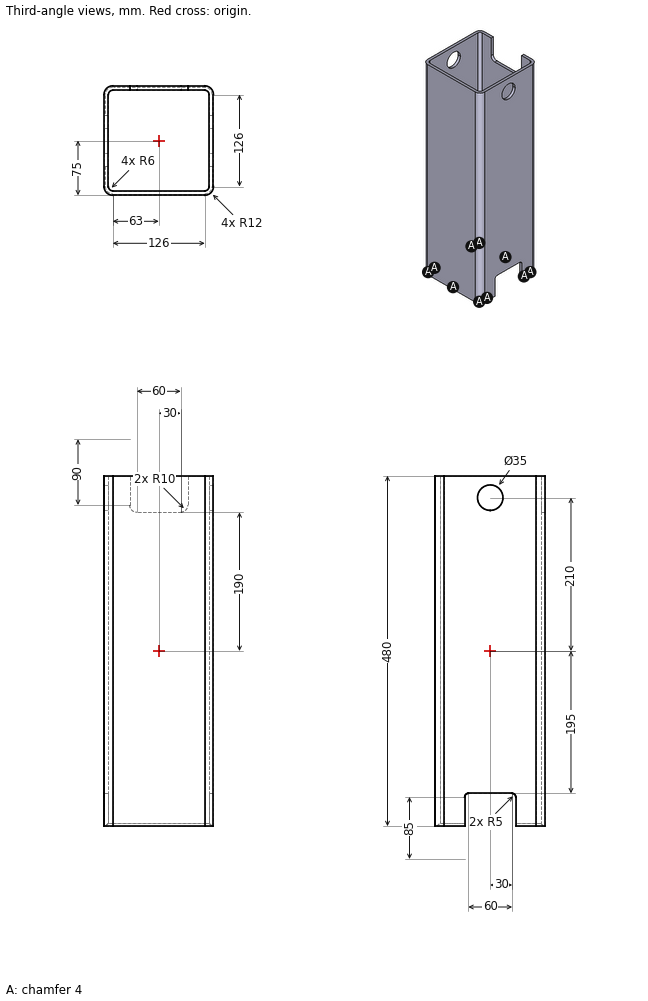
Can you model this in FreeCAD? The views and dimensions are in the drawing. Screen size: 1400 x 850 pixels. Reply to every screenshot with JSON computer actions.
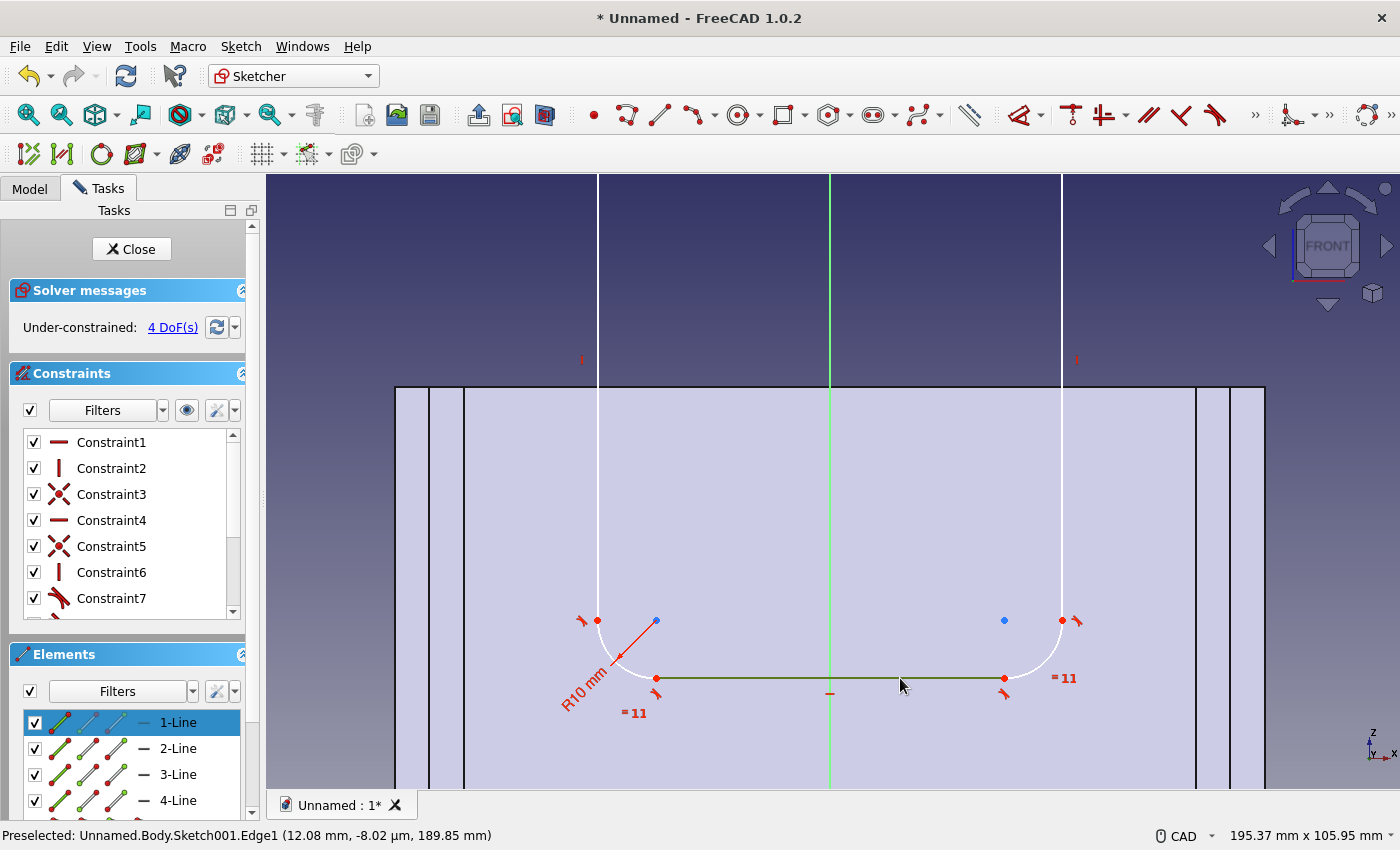
{"action": "key", "text": "l"}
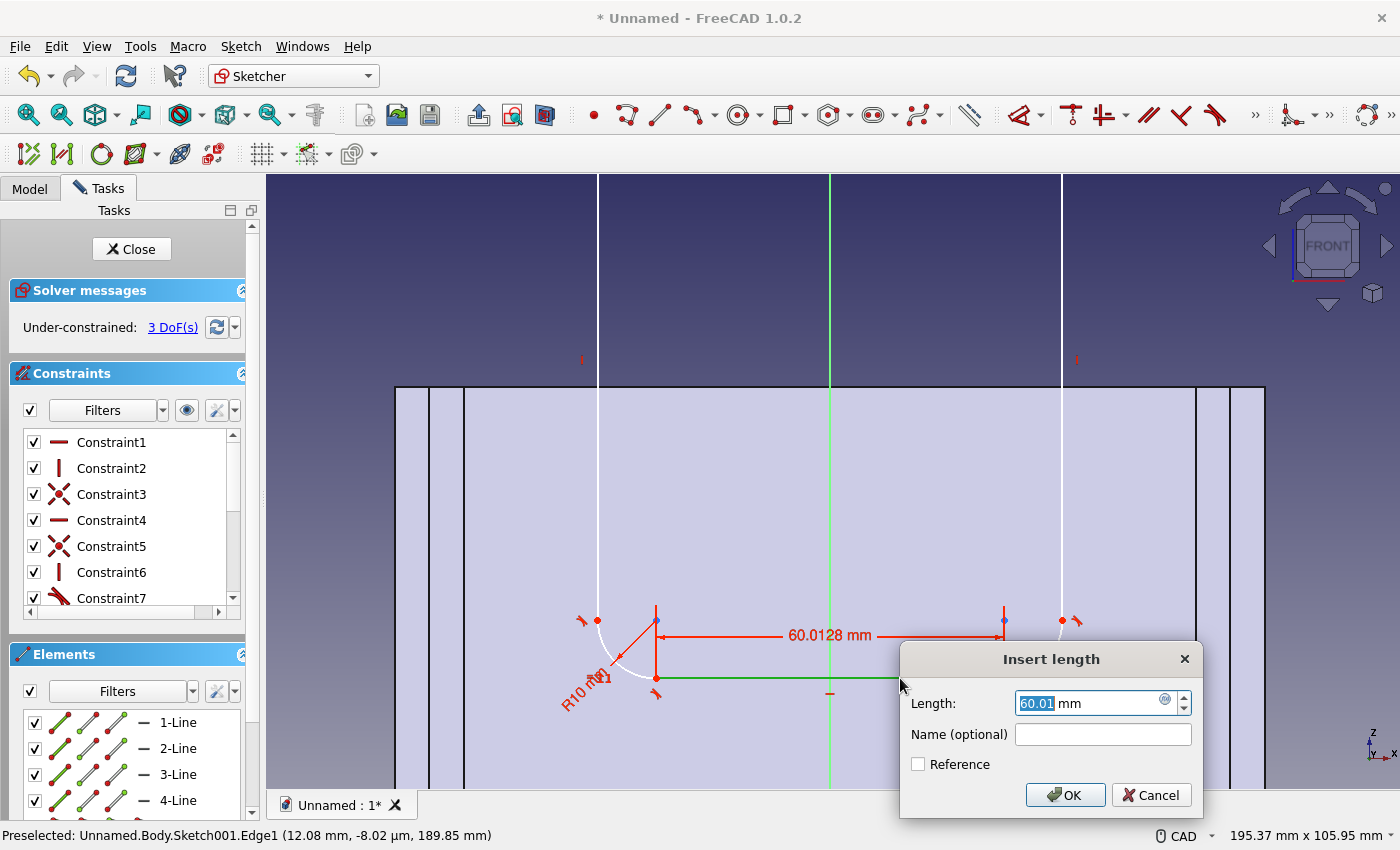
{"action": "type", "text": "60"}
{"action": "key", "text": "Return"}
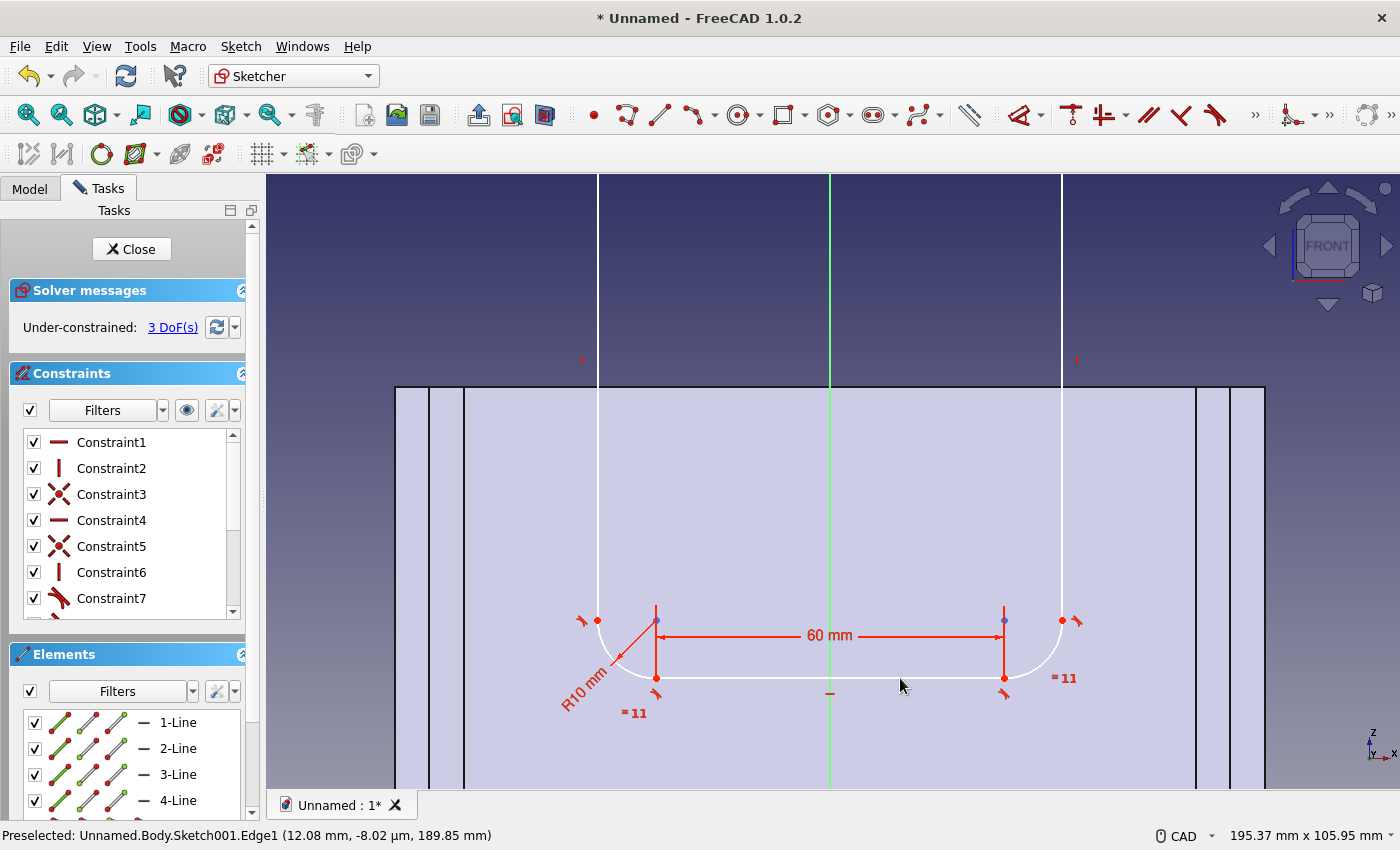
{"action": "left_click", "coordinate": [598, 464]}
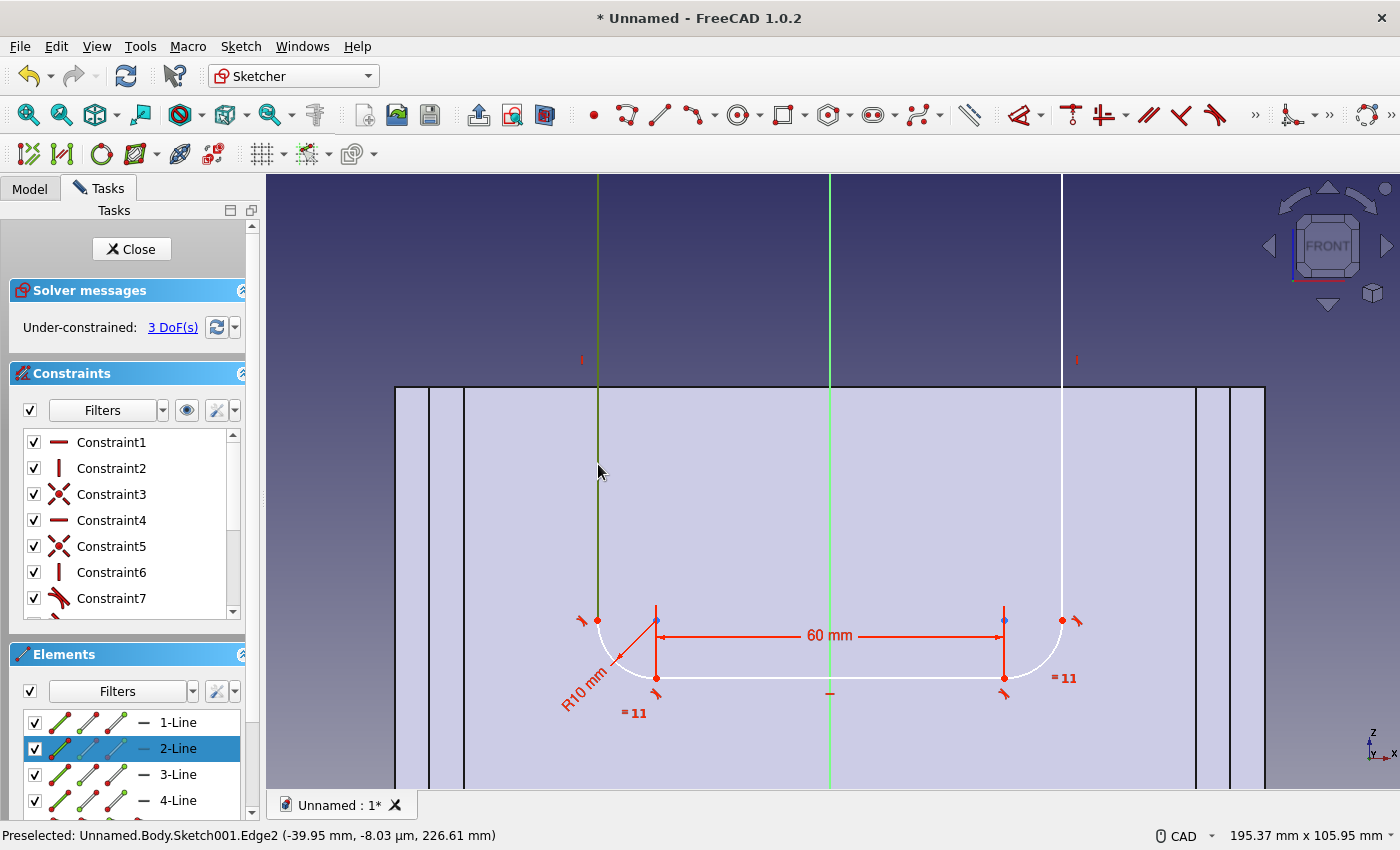
{"action": "key", "text": "i"}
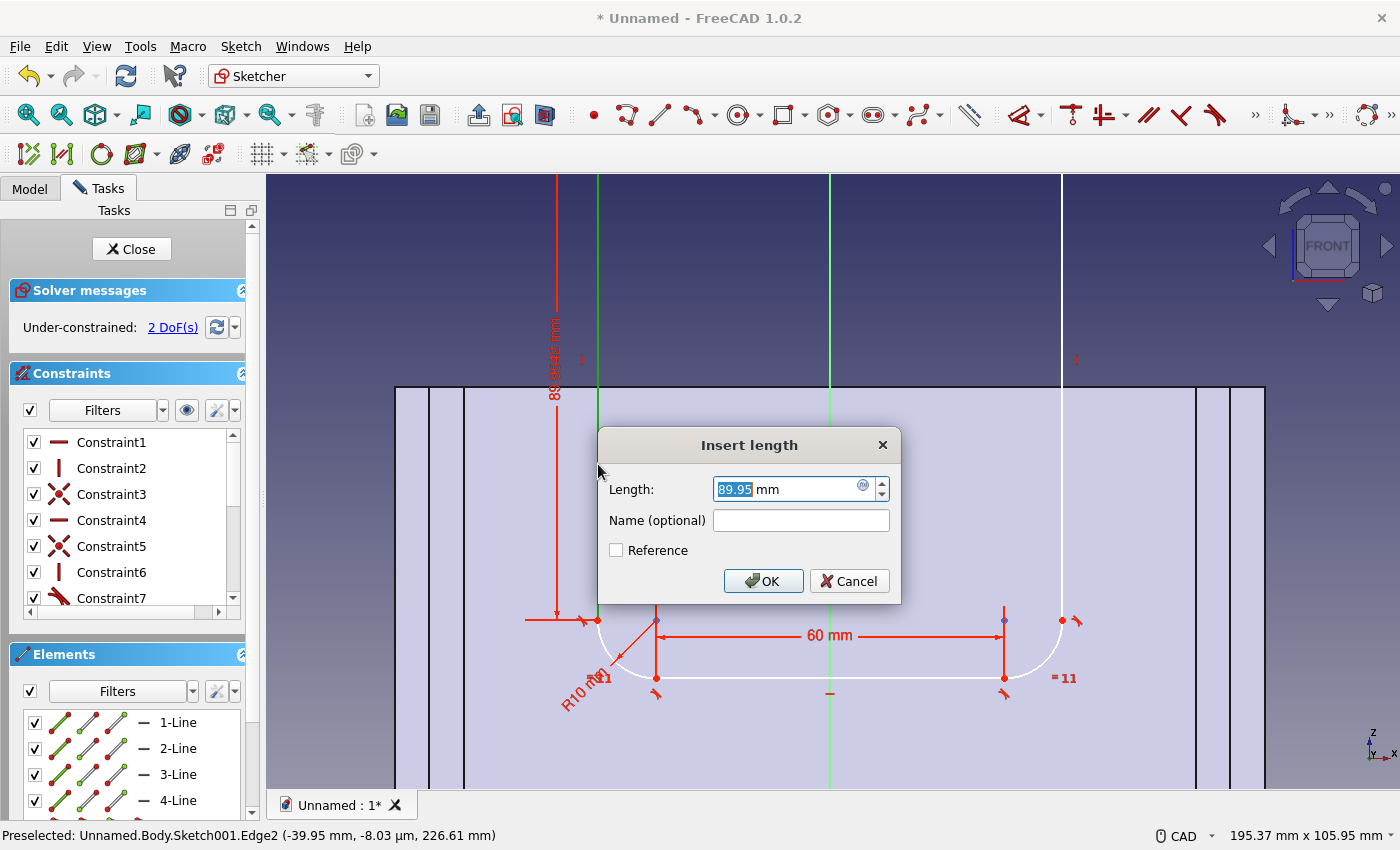
{"action": "type", "text": "90"}
{"action": "key", "text": "Return"}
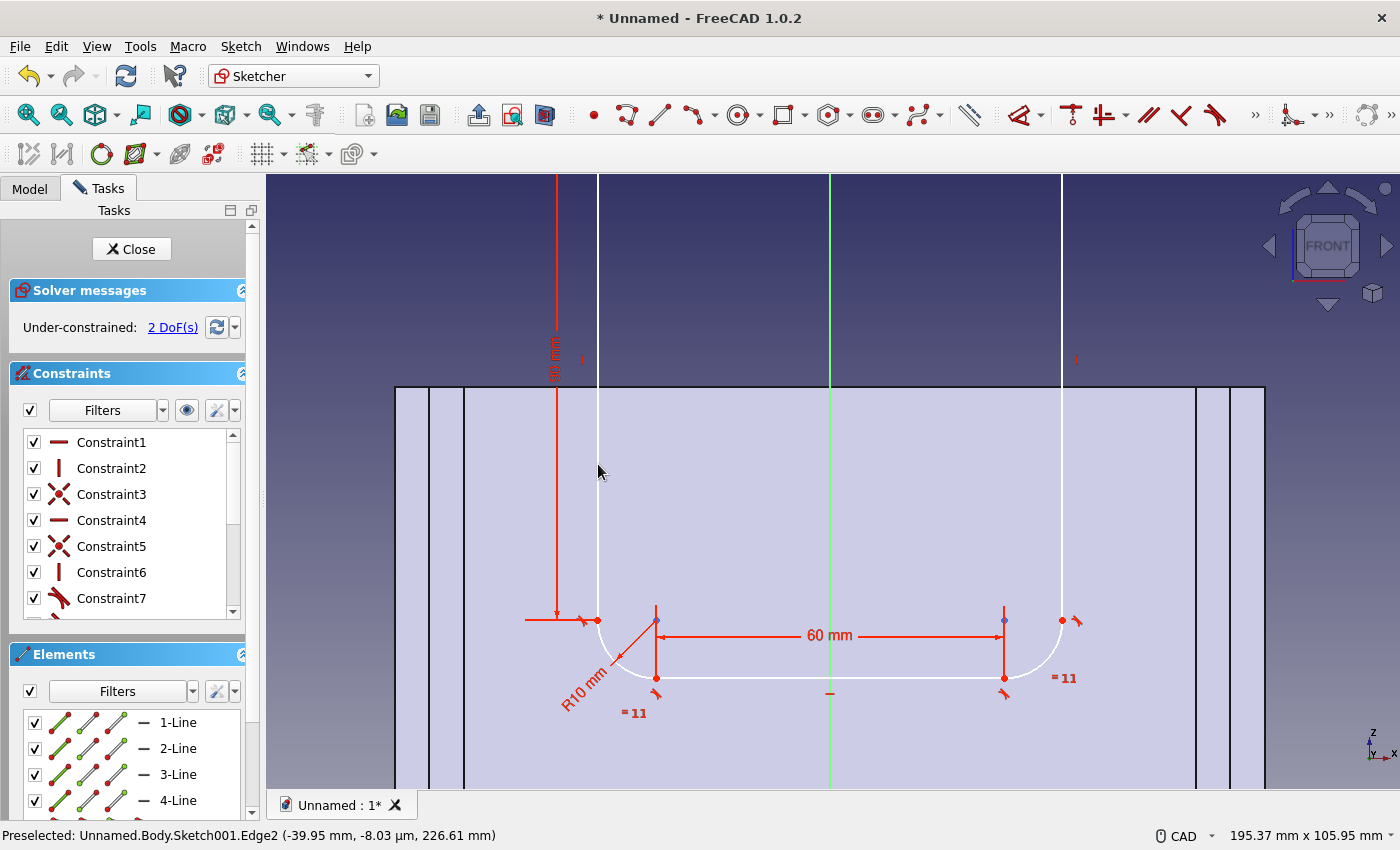
{"action": "left_click", "coordinate": [1004, 678]}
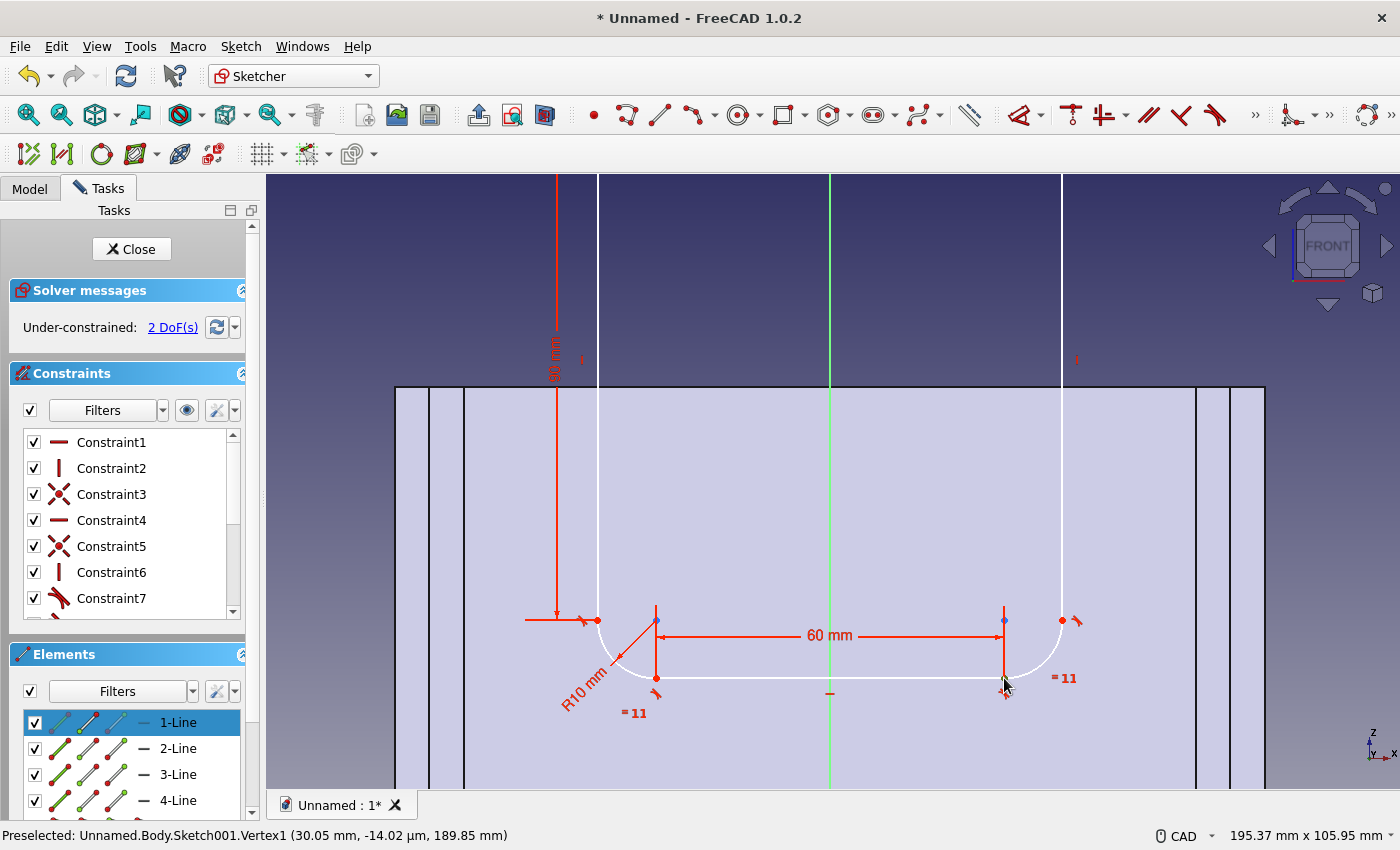
{"action": "left_click", "coordinate": [1040, 116]}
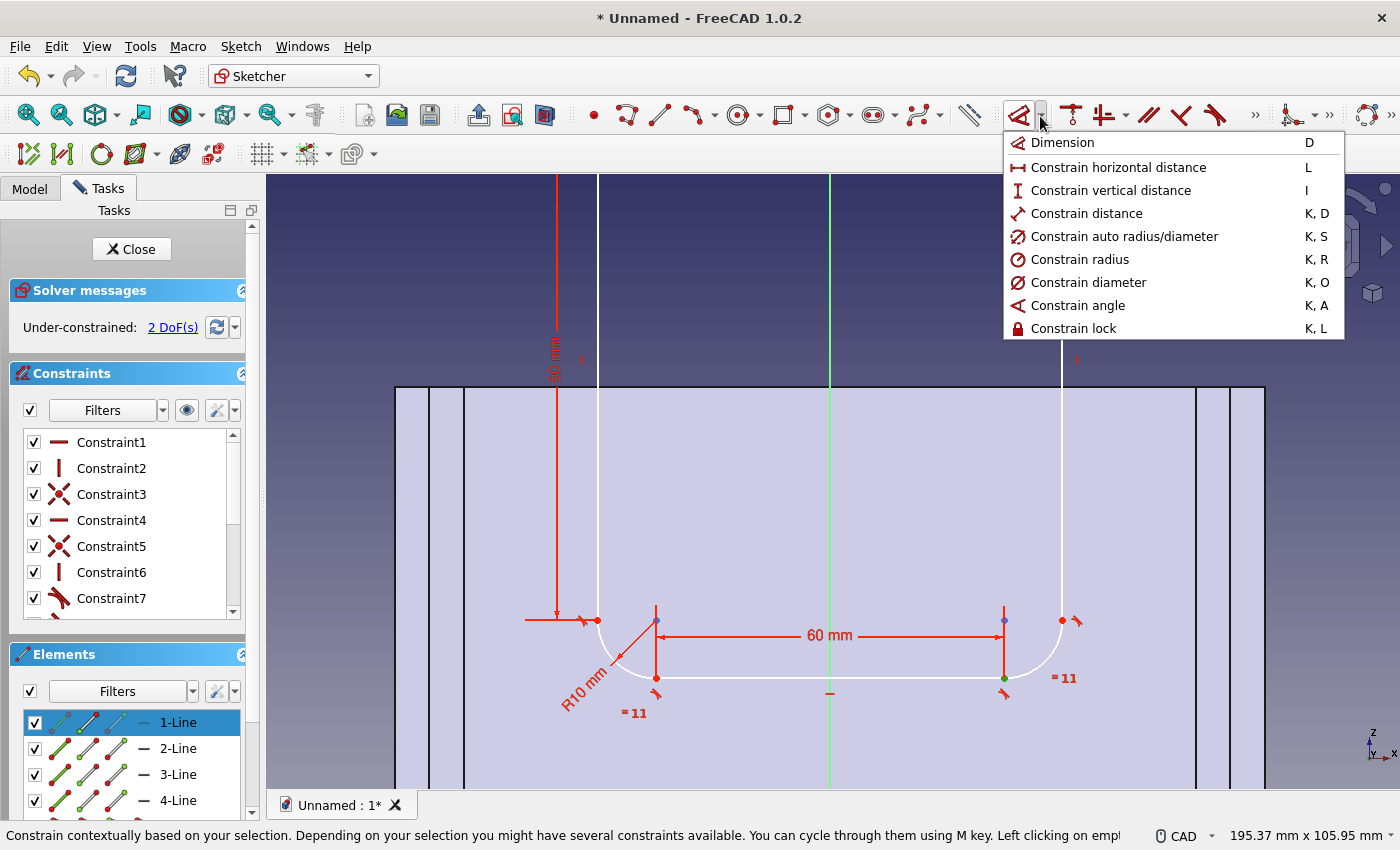
{"action": "left_click", "coordinate": [1174, 168]}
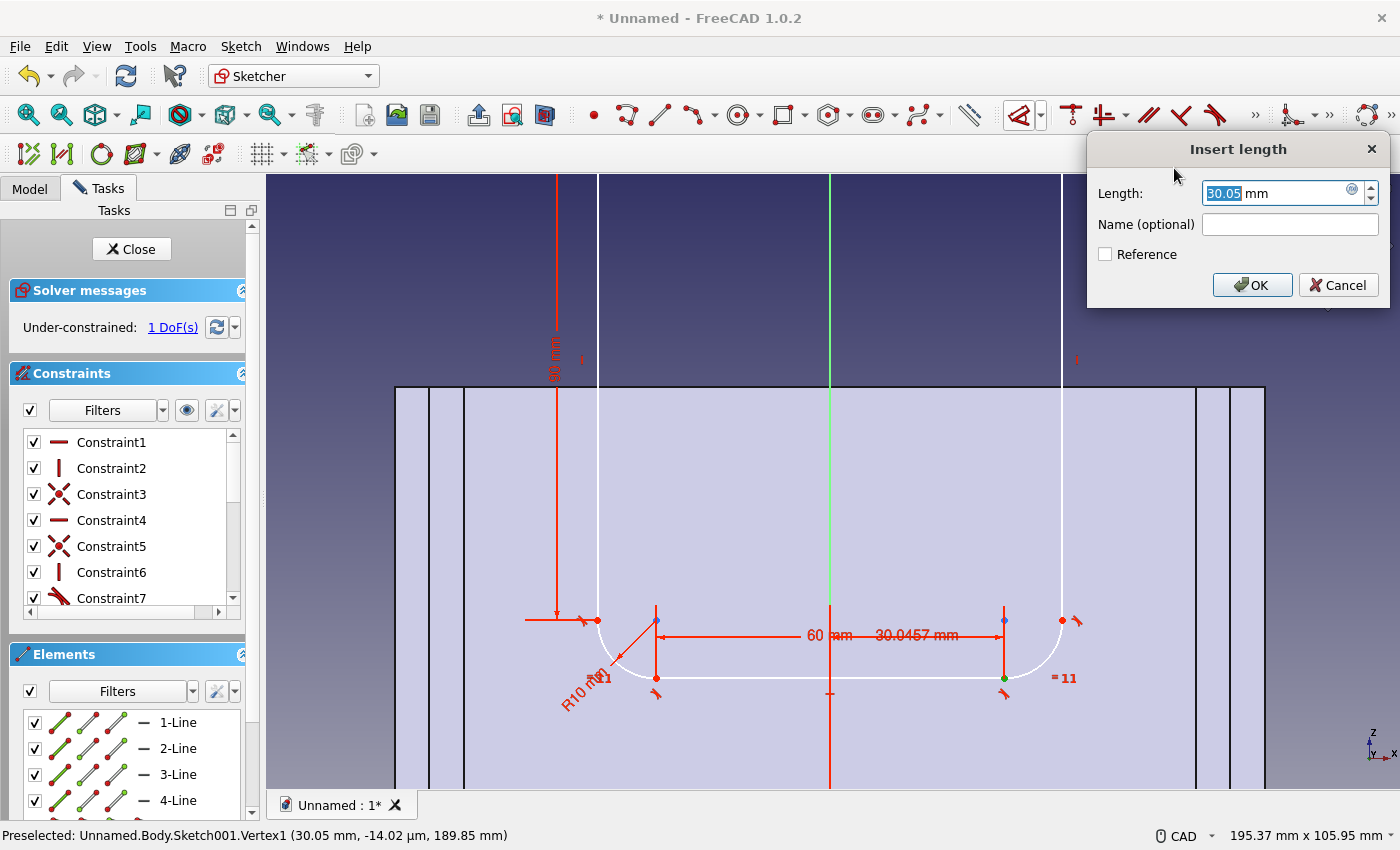
{"action": "type", "text": "30"}
{"action": "key", "text": "Return"}